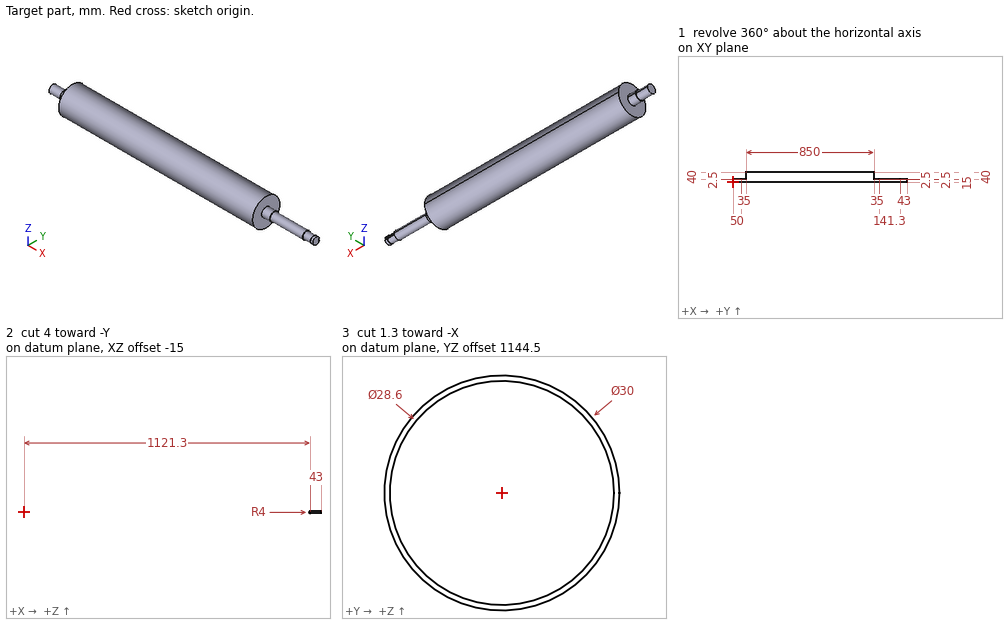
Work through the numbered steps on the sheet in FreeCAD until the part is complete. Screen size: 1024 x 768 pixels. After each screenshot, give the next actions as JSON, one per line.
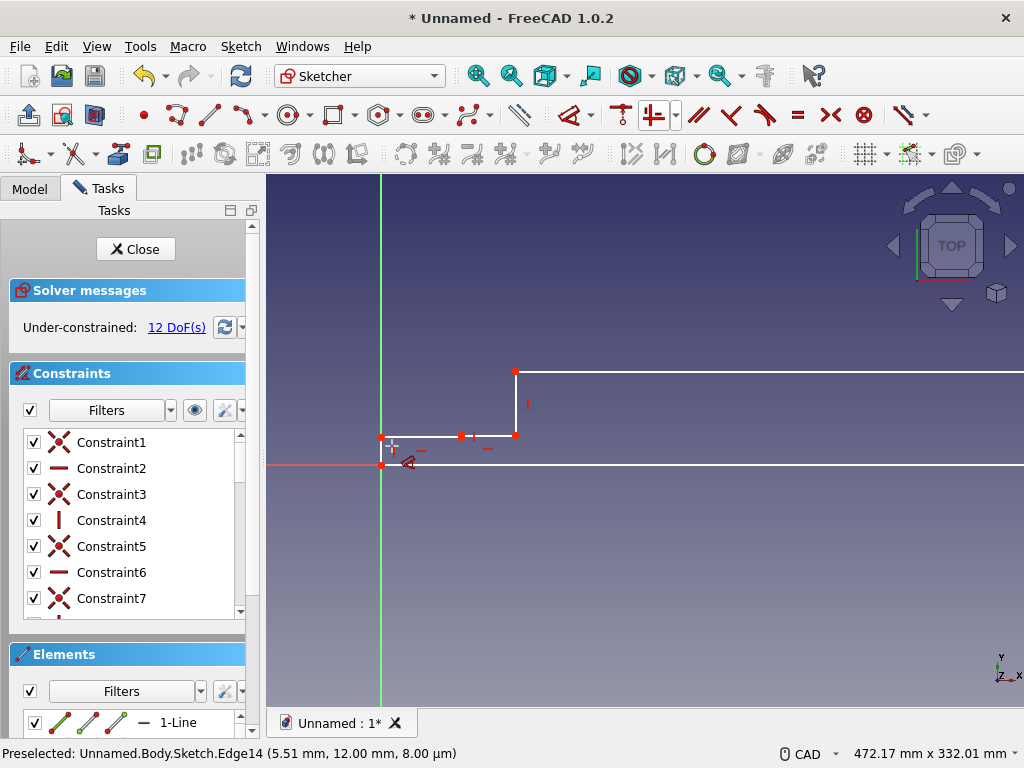
{"action": "scroll", "coordinate": [764, 449], "scroll_direction": "up", "scroll_amount": 12}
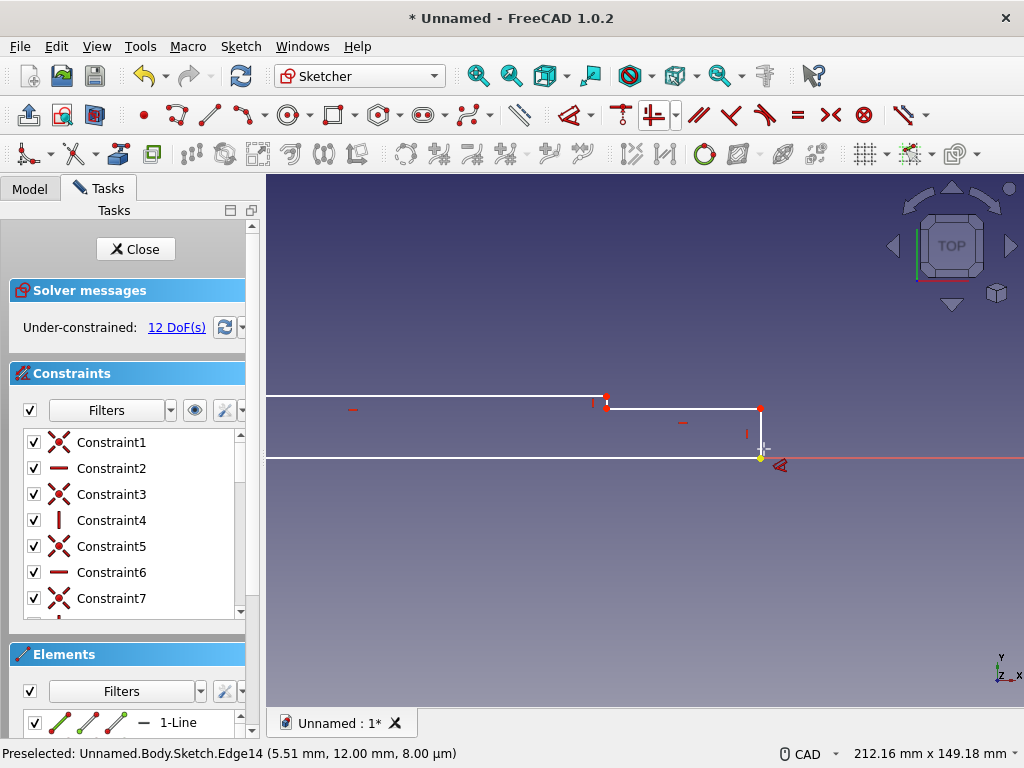
{"action": "left_click", "coordinate": [761, 444]}
{"action": "left_click", "coordinate": [795, 434]}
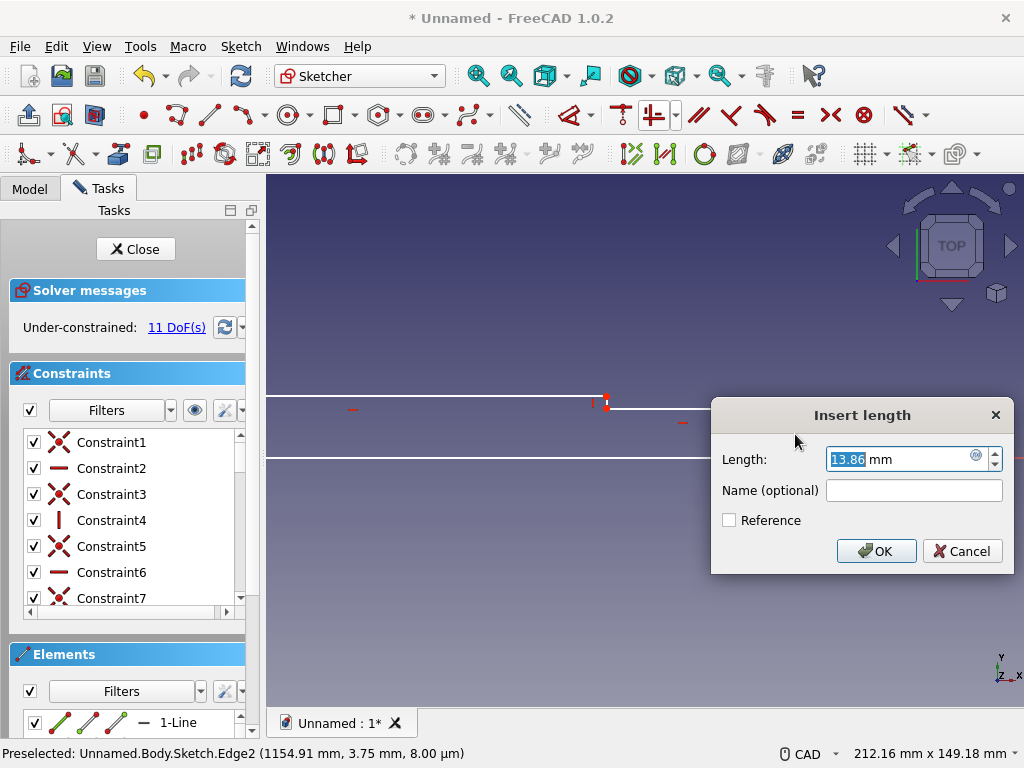
{"action": "type", "text": "15"}
{"action": "key", "text": "Return"}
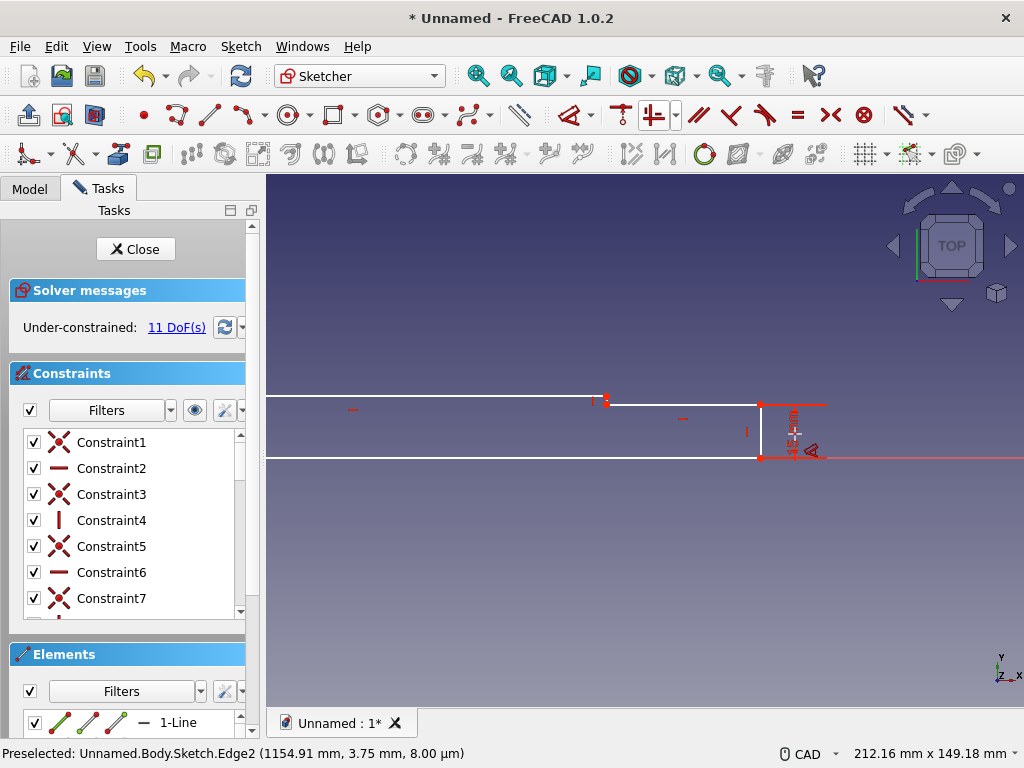
{"action": "scroll", "coordinate": [764, 449], "scroll_direction": "down", "scroll_amount": 12}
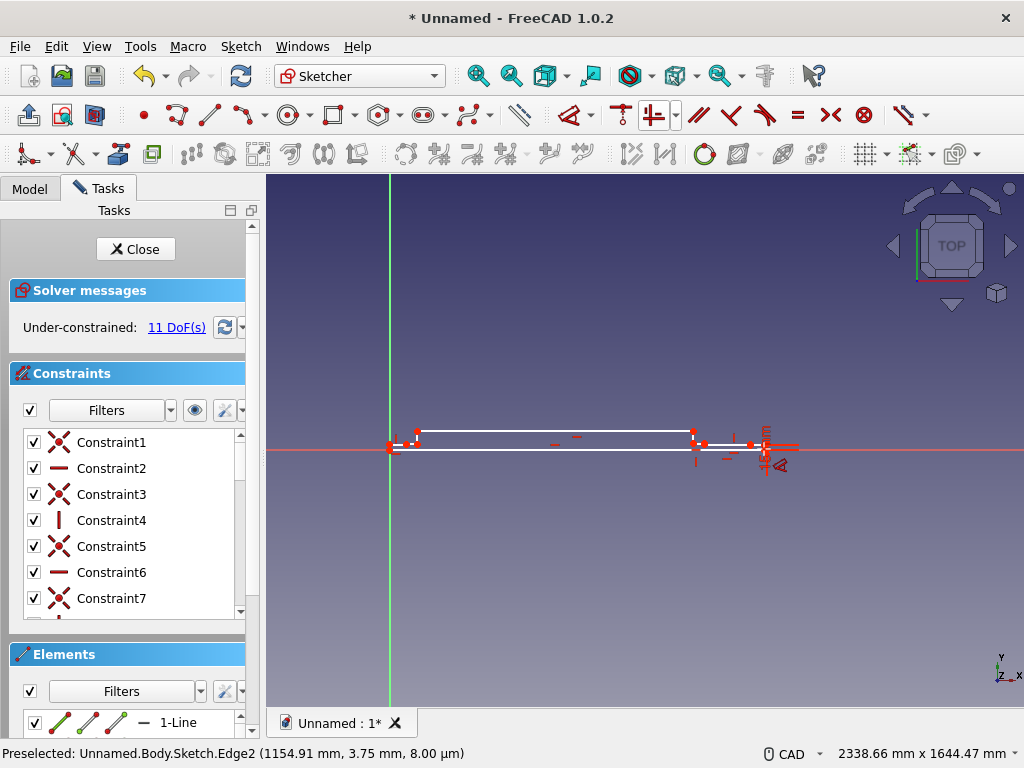
{"action": "scroll", "coordinate": [760, 445], "scroll_direction": "up", "scroll_amount": 6}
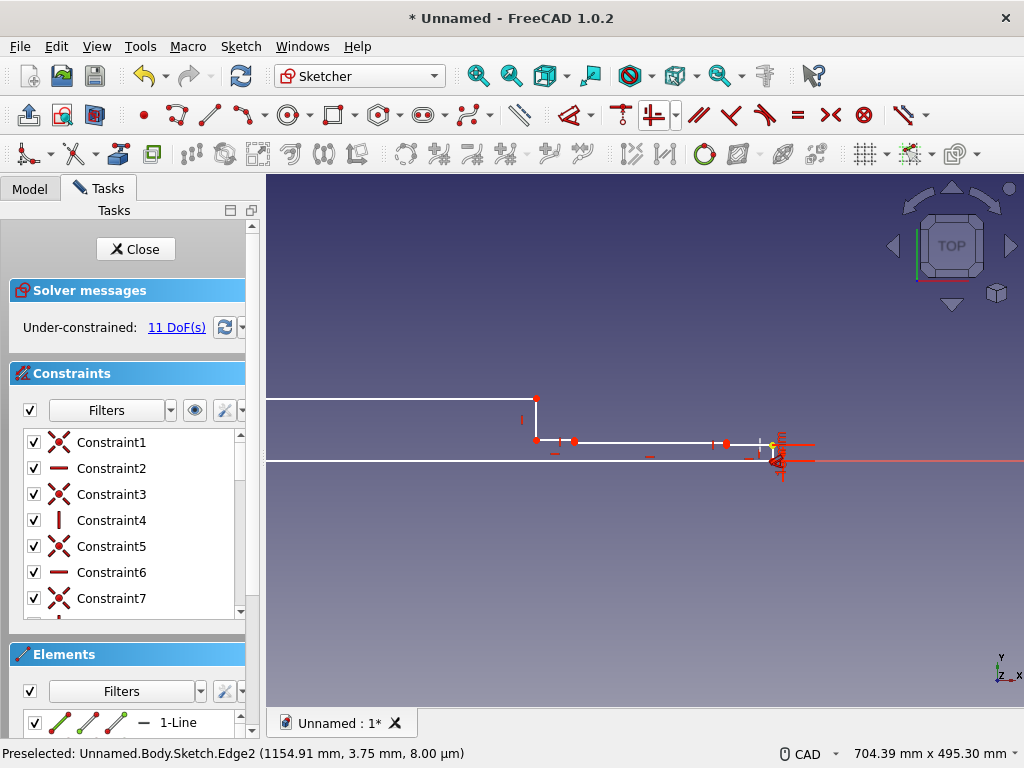
{"action": "left_click", "coordinate": [759, 445]}
{"action": "left_click", "coordinate": [750, 479]}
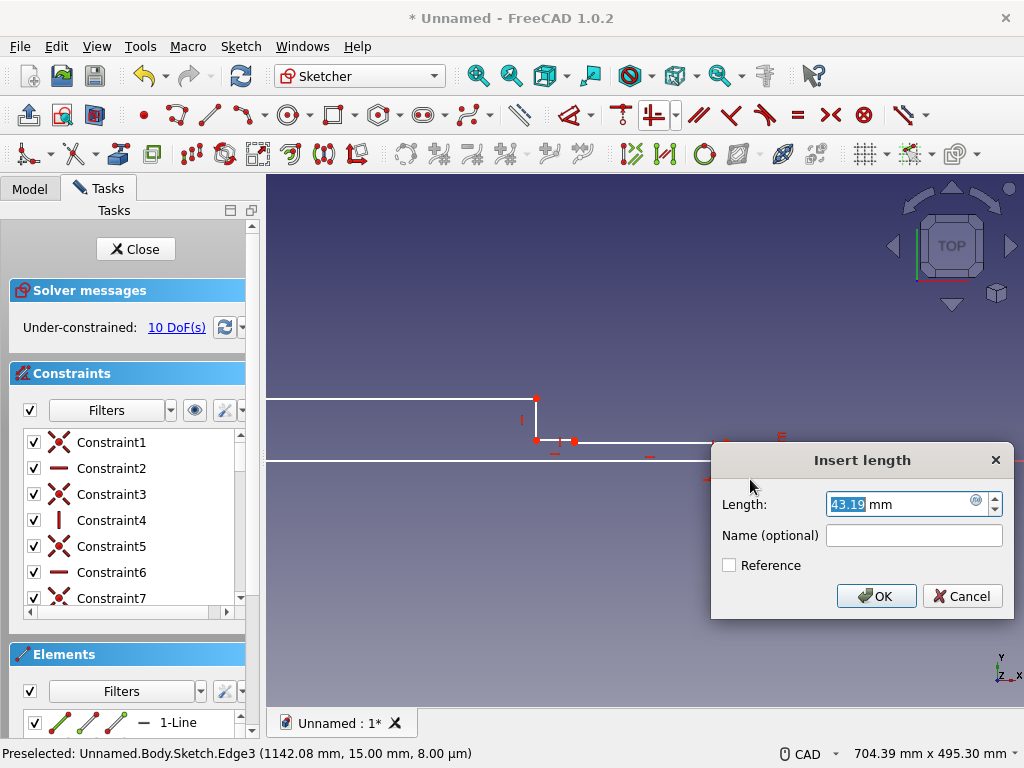
{"action": "type", "text": "43"}
{"action": "key", "text": "Return"}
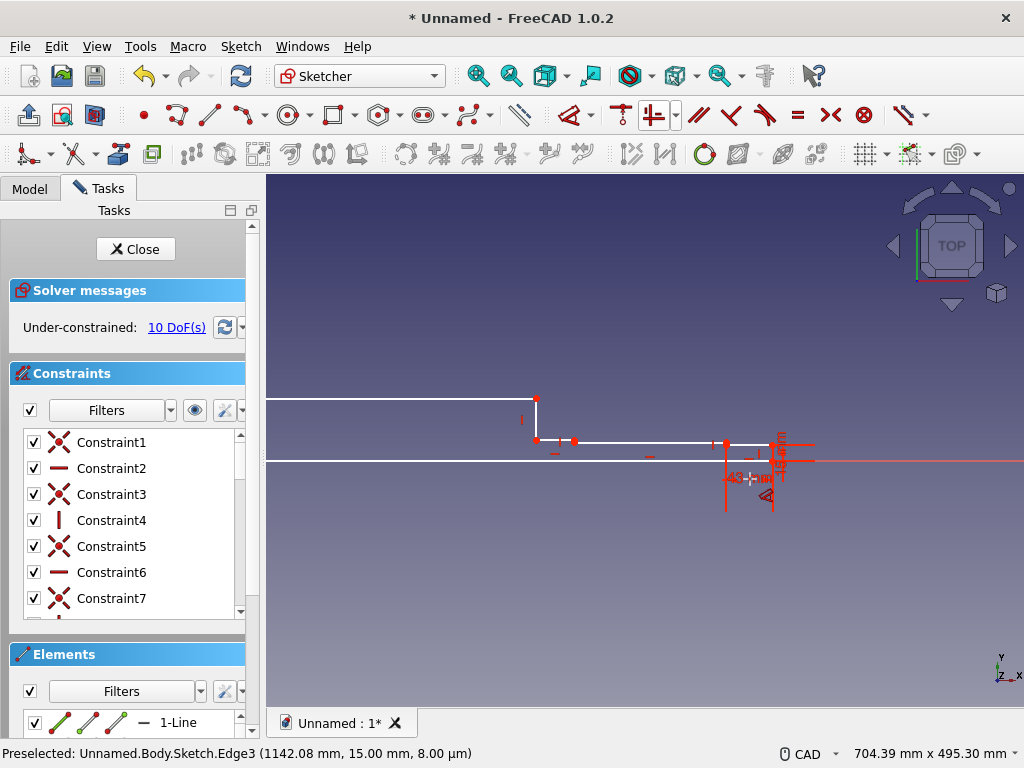
{"action": "left_click", "coordinate": [563, 440]}
{"action": "left_click", "coordinate": [555, 406]}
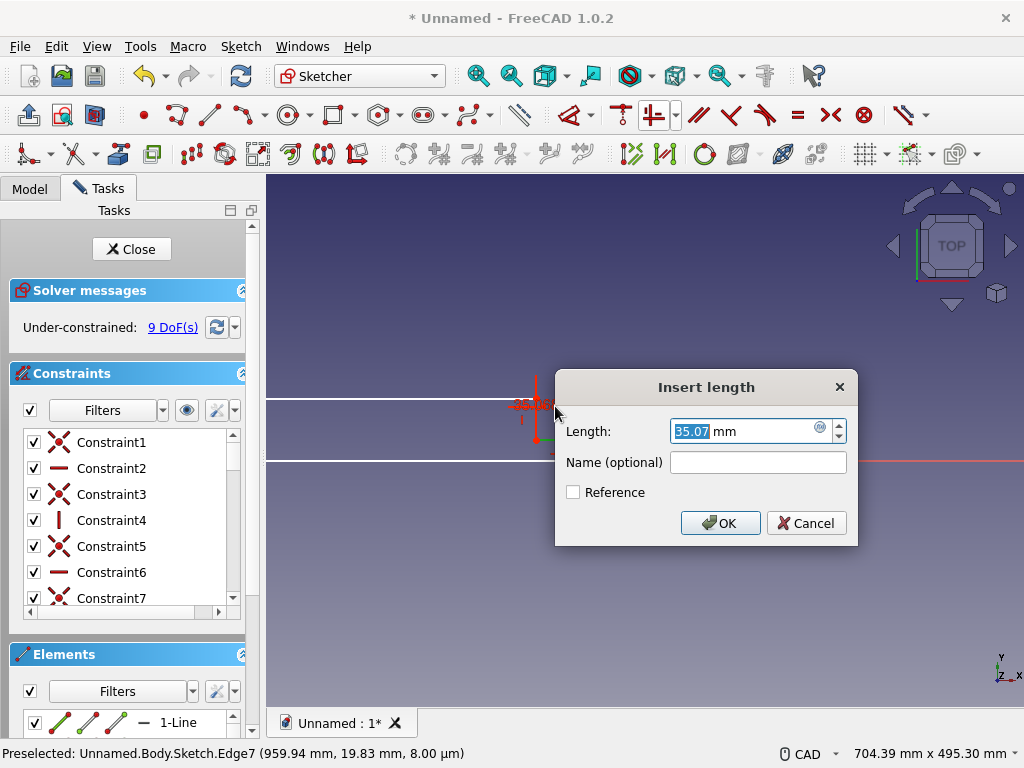
{"action": "type", "text": "35"}
{"action": "key", "text": "Return"}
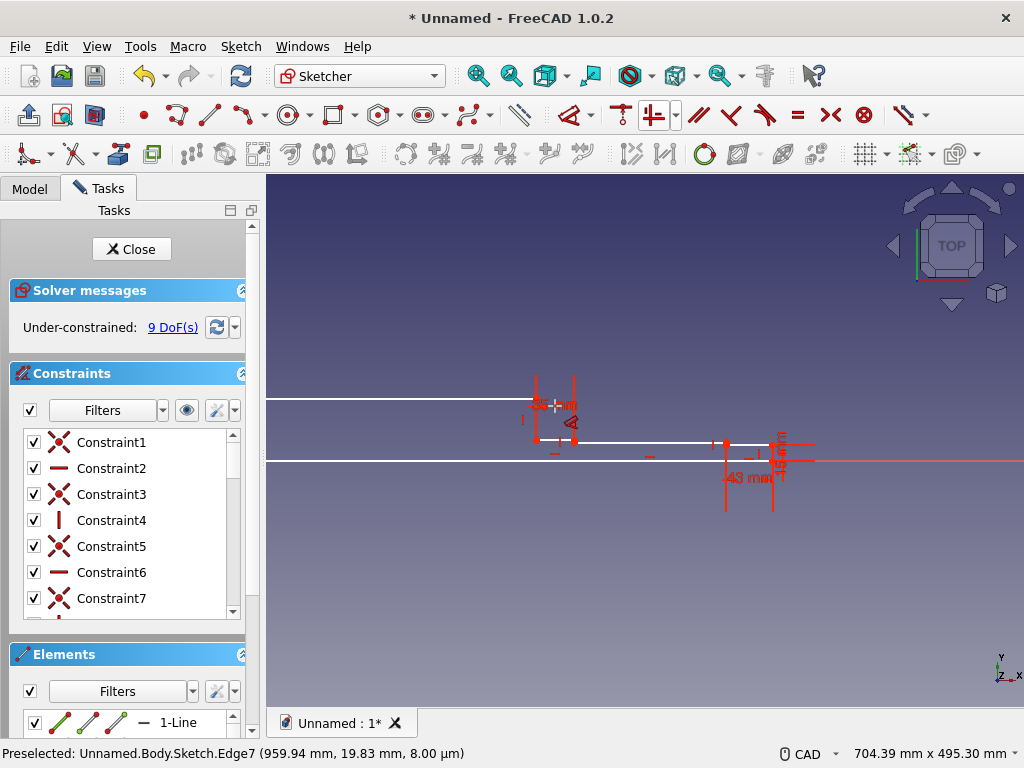
{"action": "left_click", "coordinate": [536, 428]}
{"action": "left_click", "coordinate": [502, 429]}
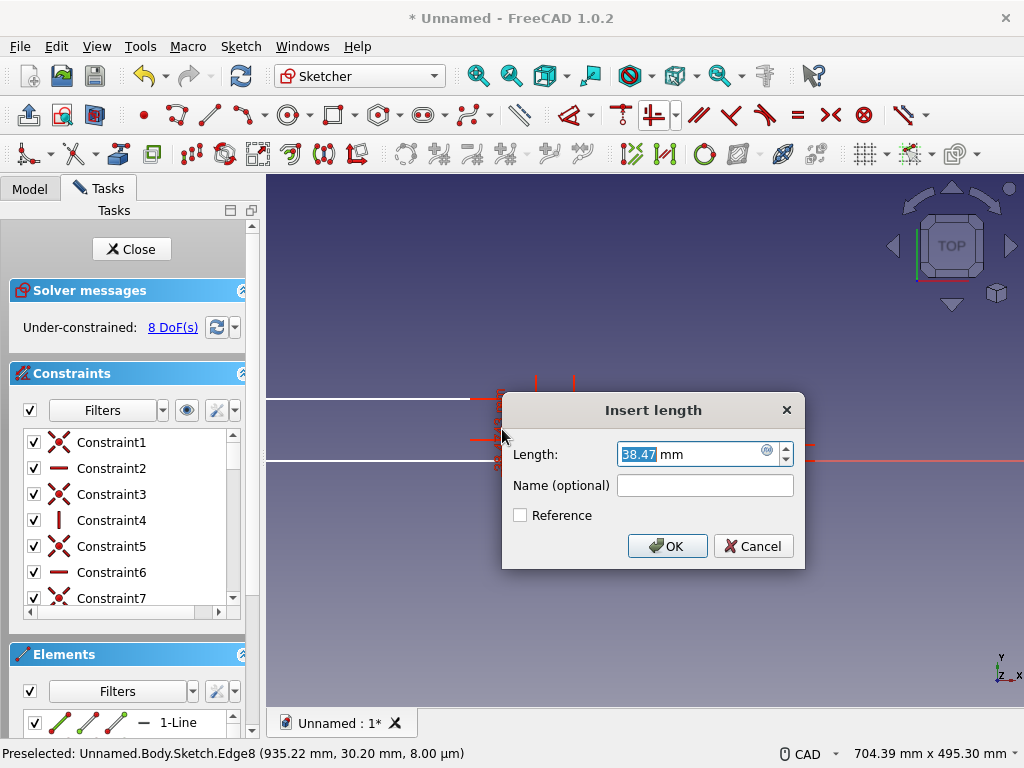
{"action": "type", "text": "40"}
{"action": "key", "text": "Return"}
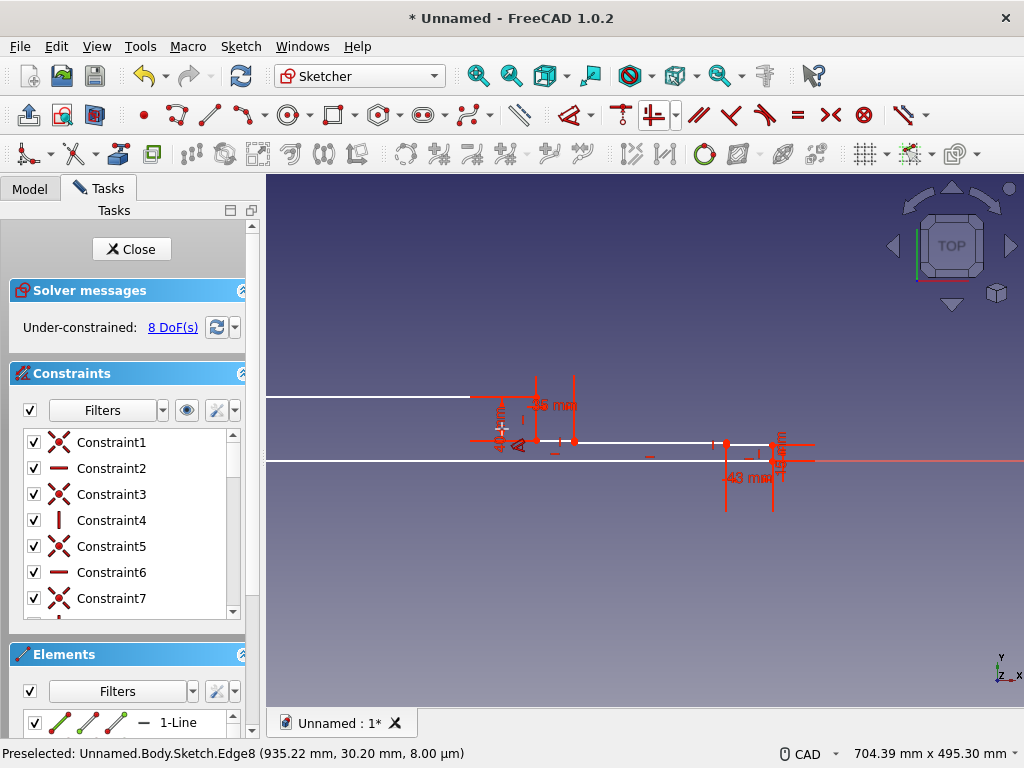
{"action": "scroll", "coordinate": [760, 445], "scroll_direction": "down", "scroll_amount": 6}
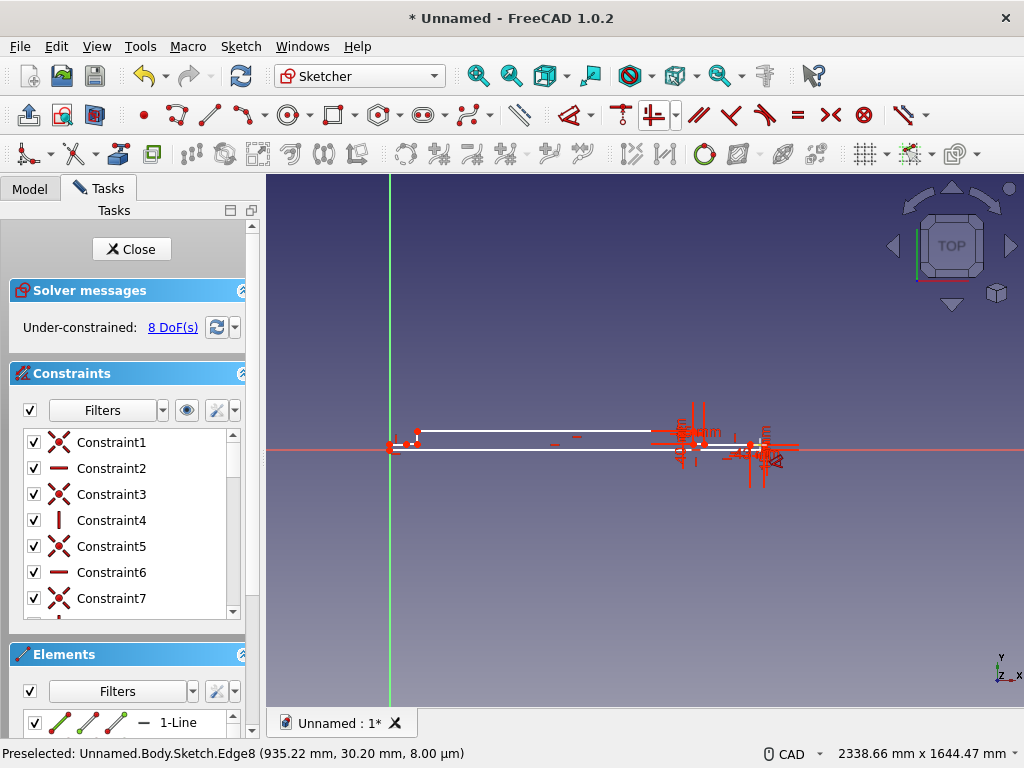
{"action": "scroll", "coordinate": [417, 435], "scroll_direction": "up", "scroll_amount": 7}